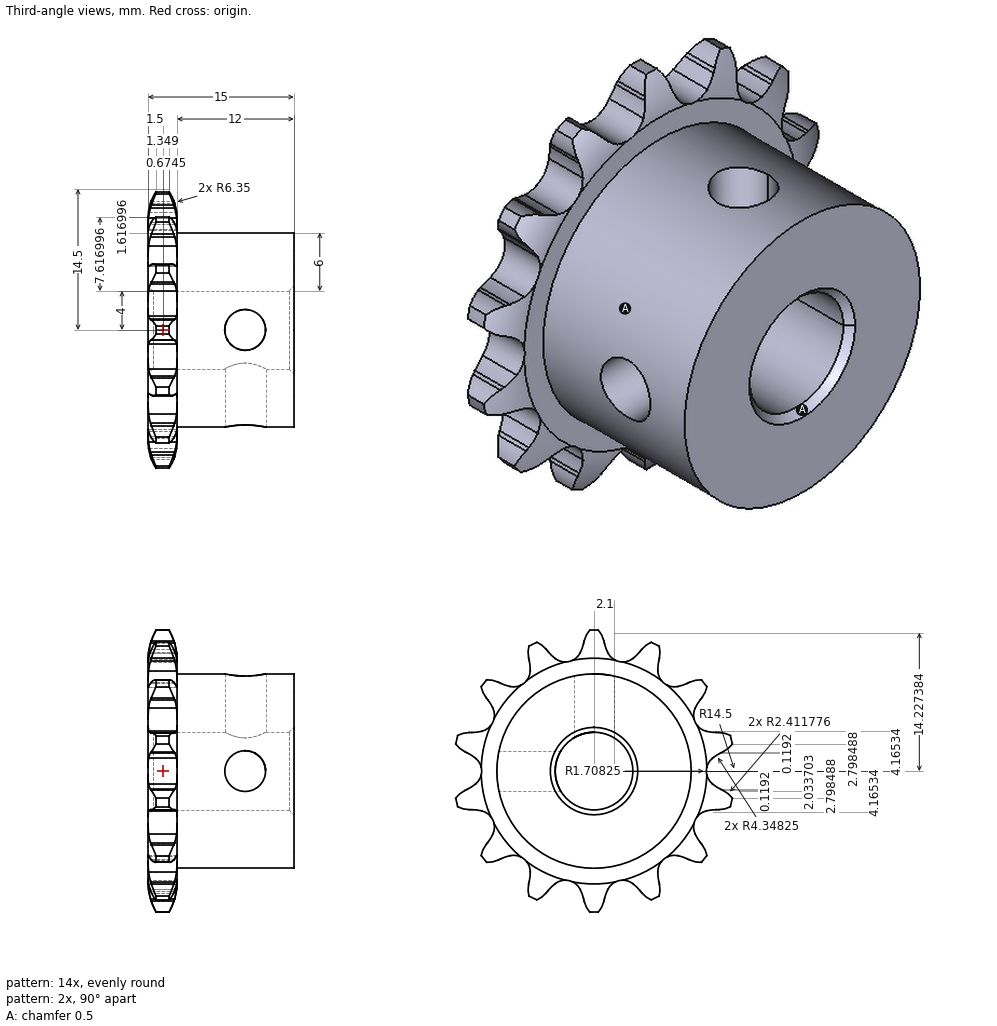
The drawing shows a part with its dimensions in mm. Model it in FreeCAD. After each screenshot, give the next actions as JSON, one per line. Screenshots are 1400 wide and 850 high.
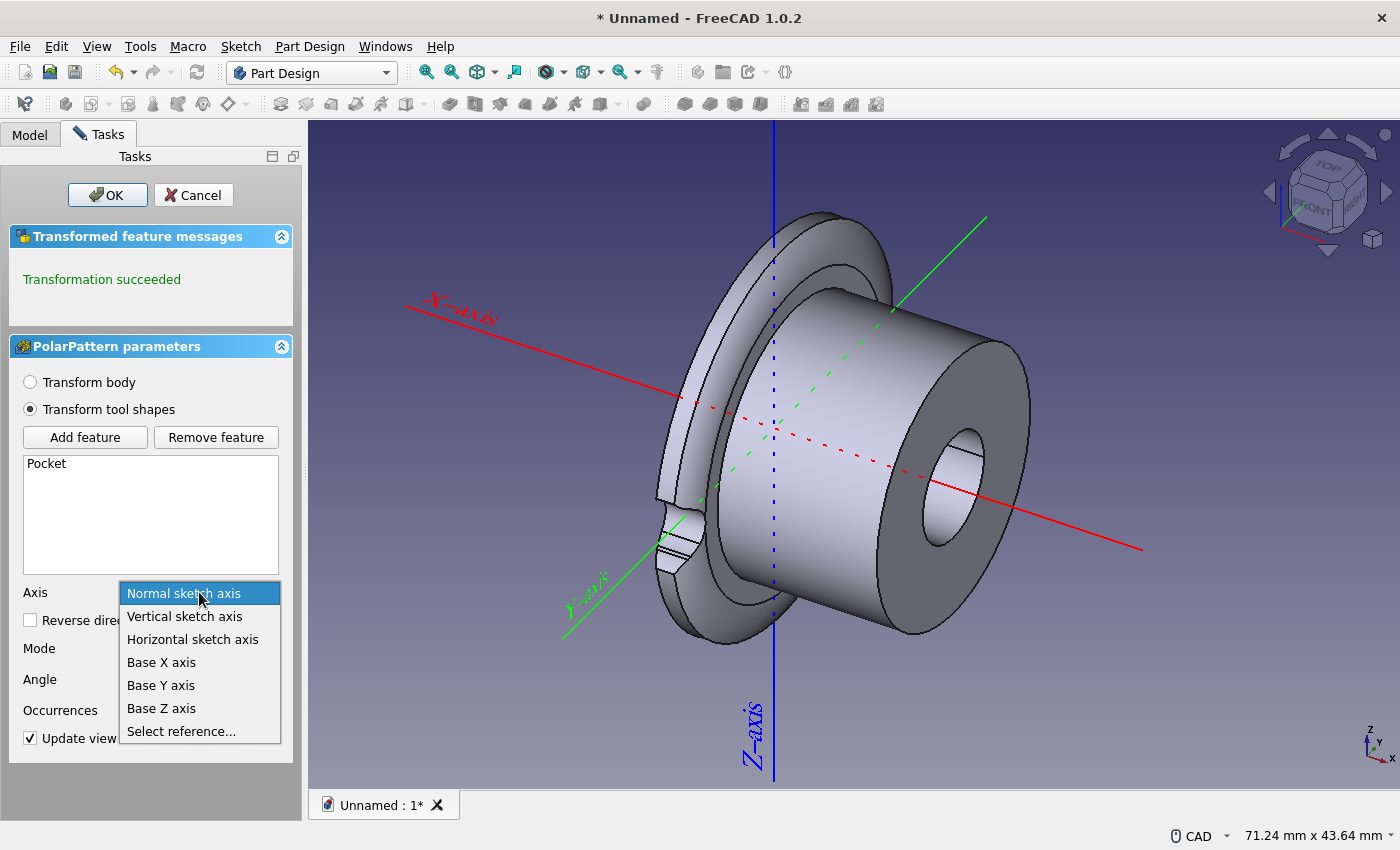
{"action": "left_click", "coordinate": [198, 662]}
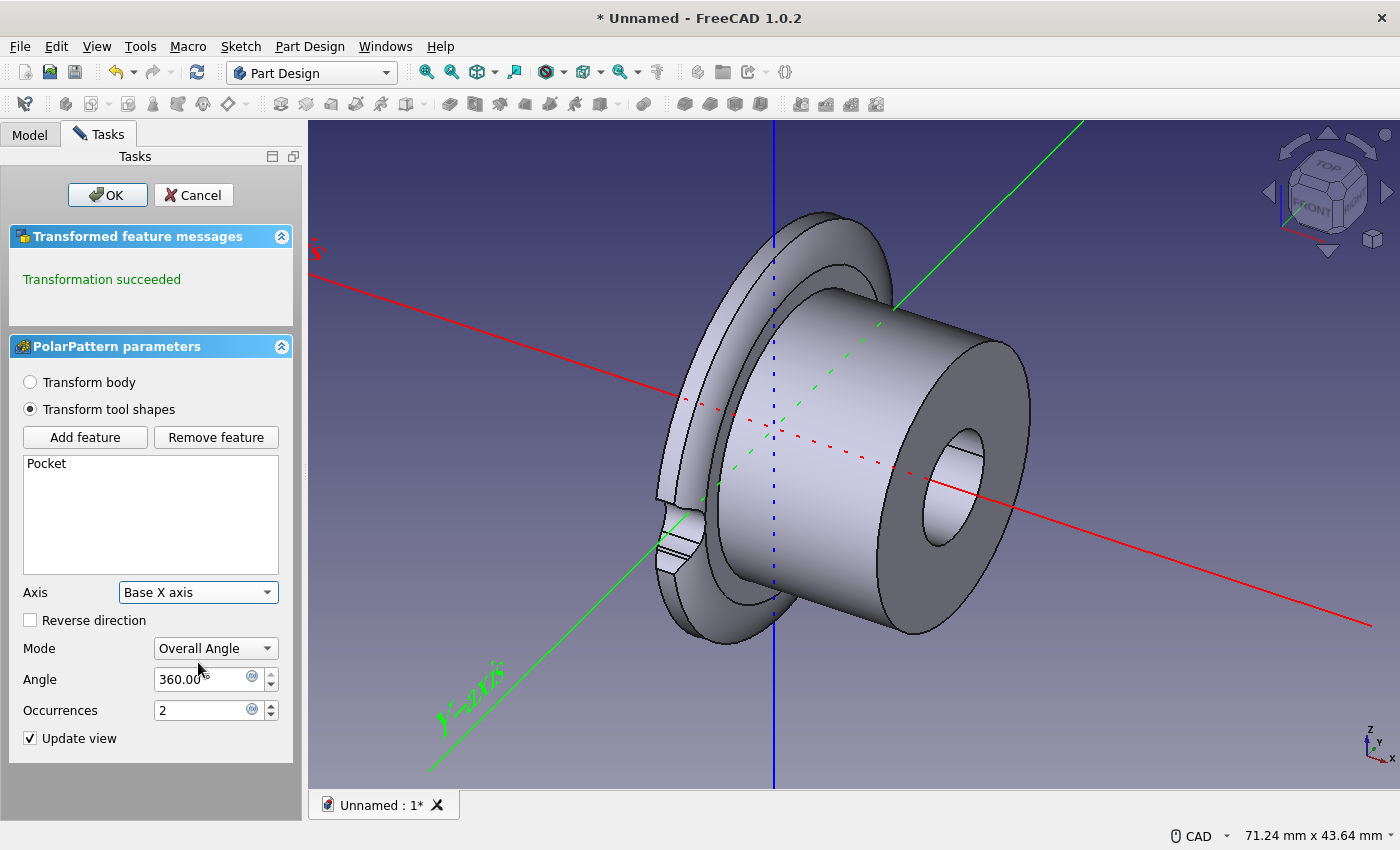
{"action": "triple_click", "coordinate": [210, 710]}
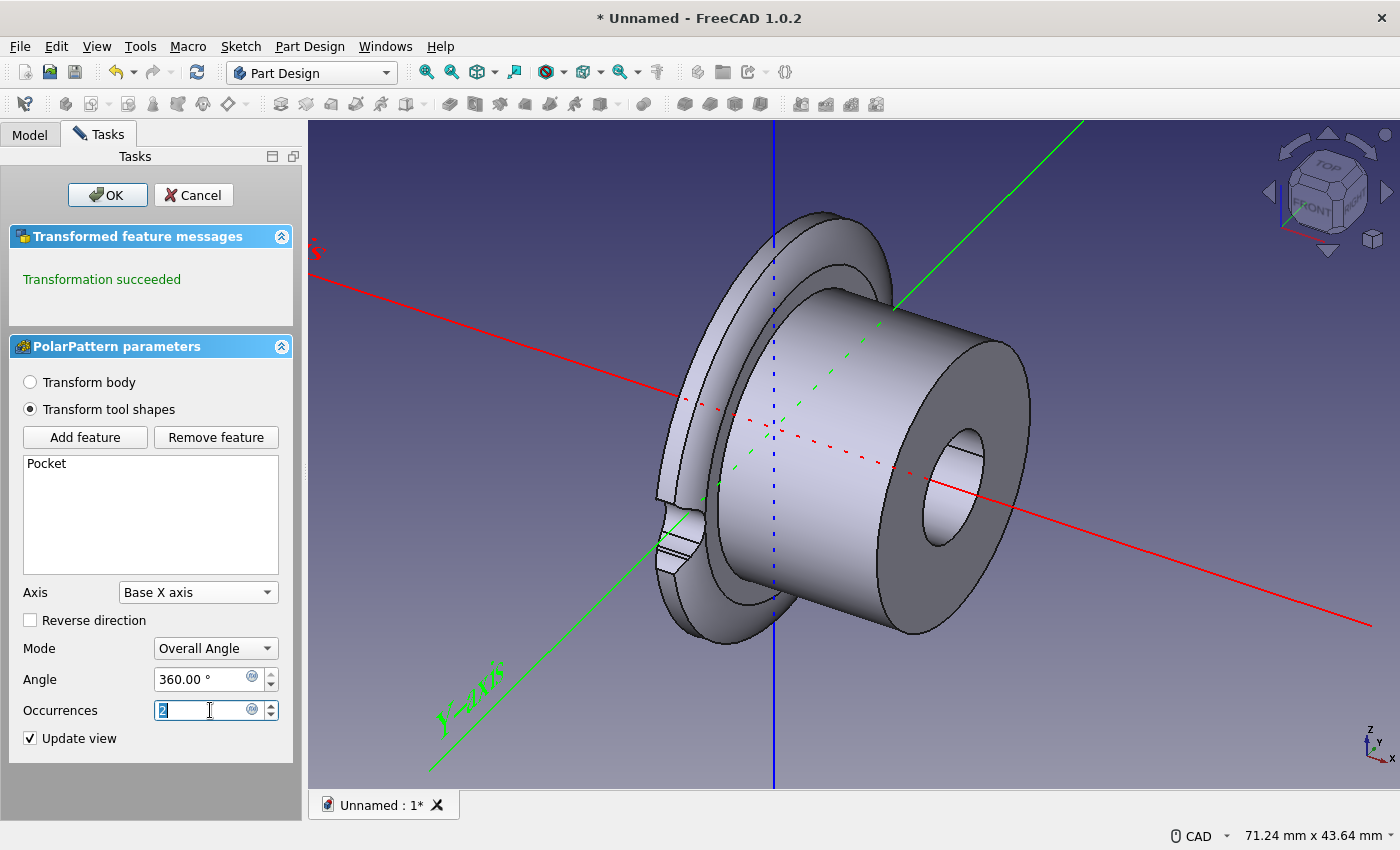
{"action": "type", "text": "14"}
{"action": "key", "text": "Tab"}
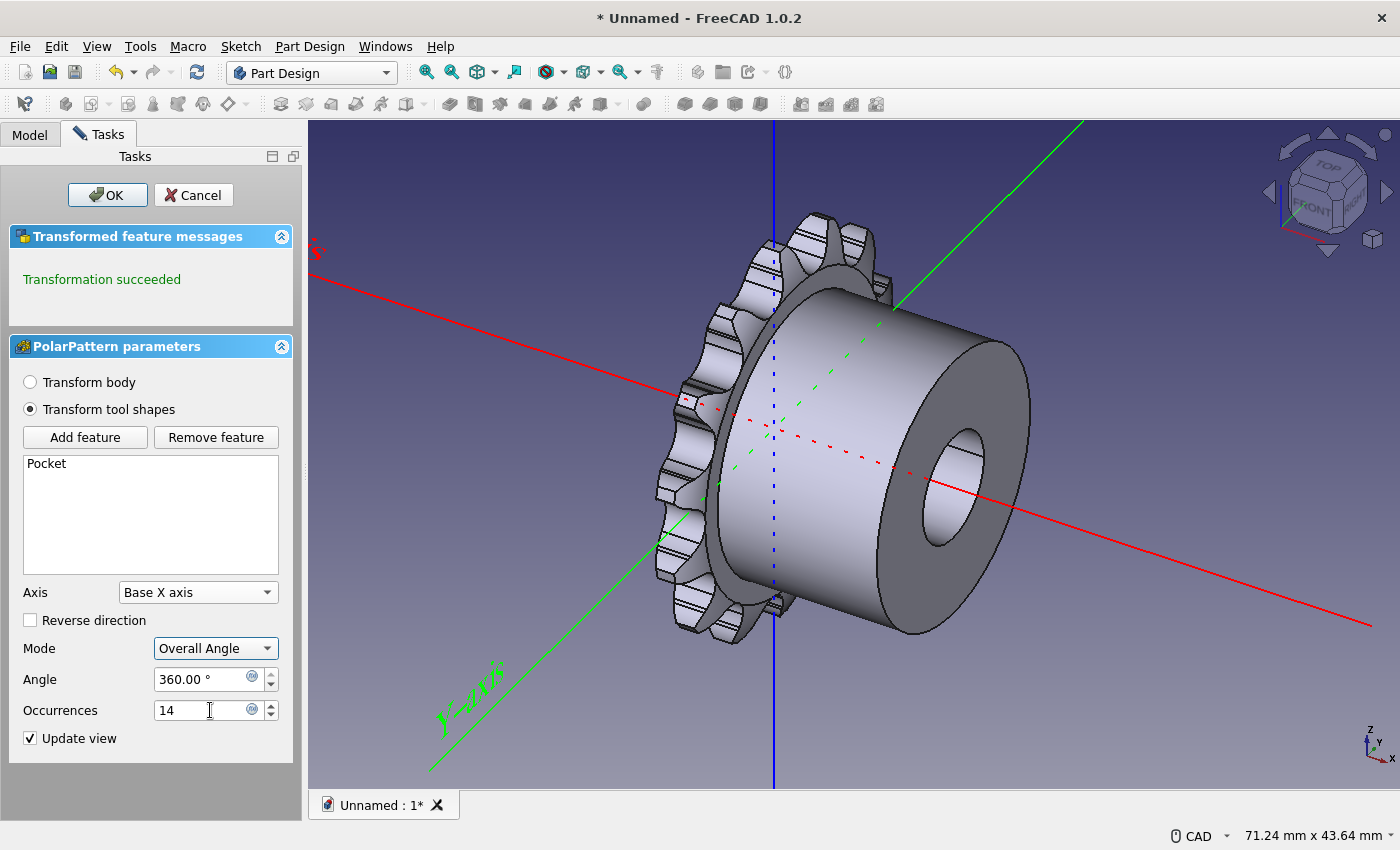
{"action": "left_click", "coordinate": [108, 195]}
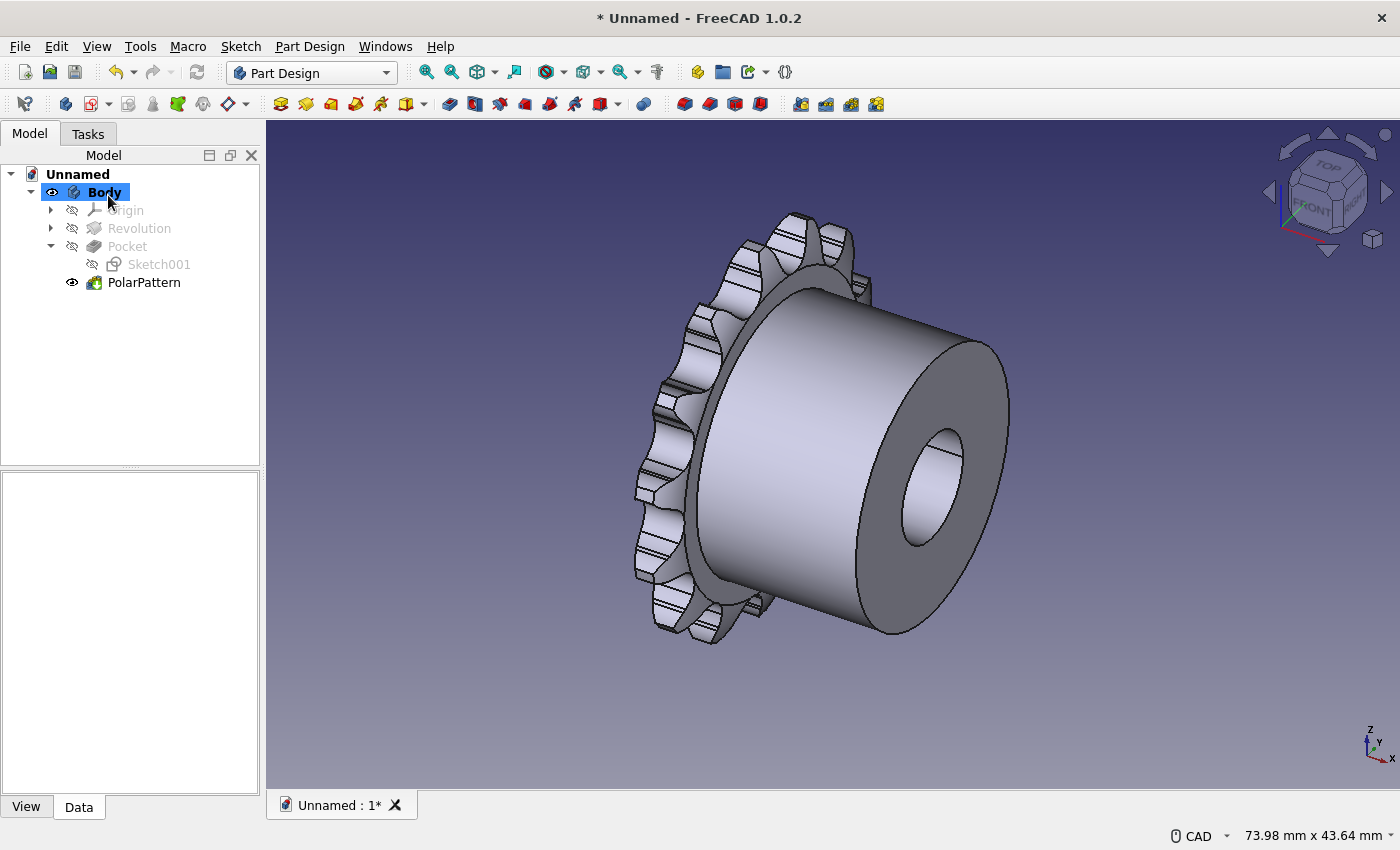
{"action": "left_click", "coordinate": [51, 210]}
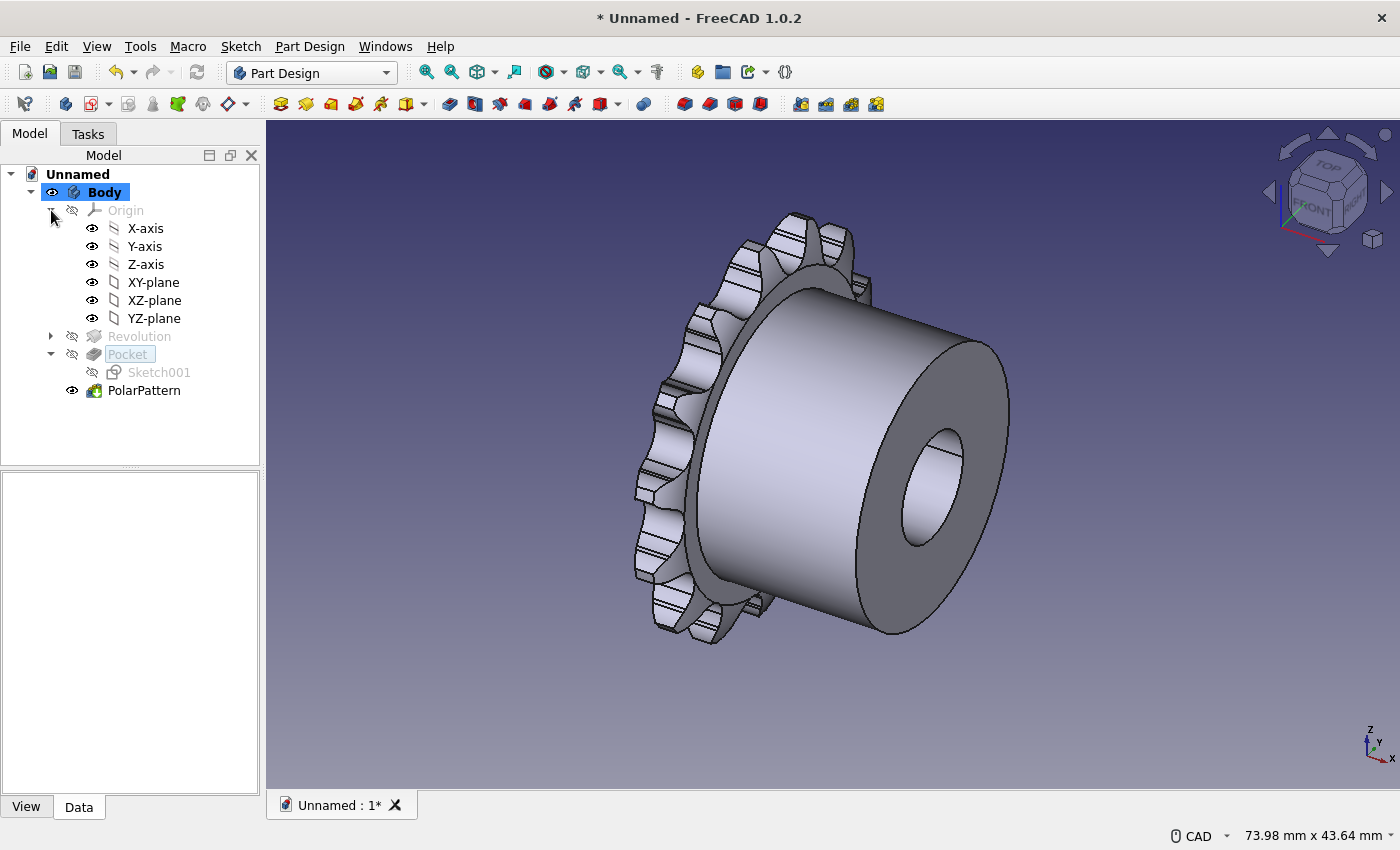
{"action": "left_click", "coordinate": [137, 318]}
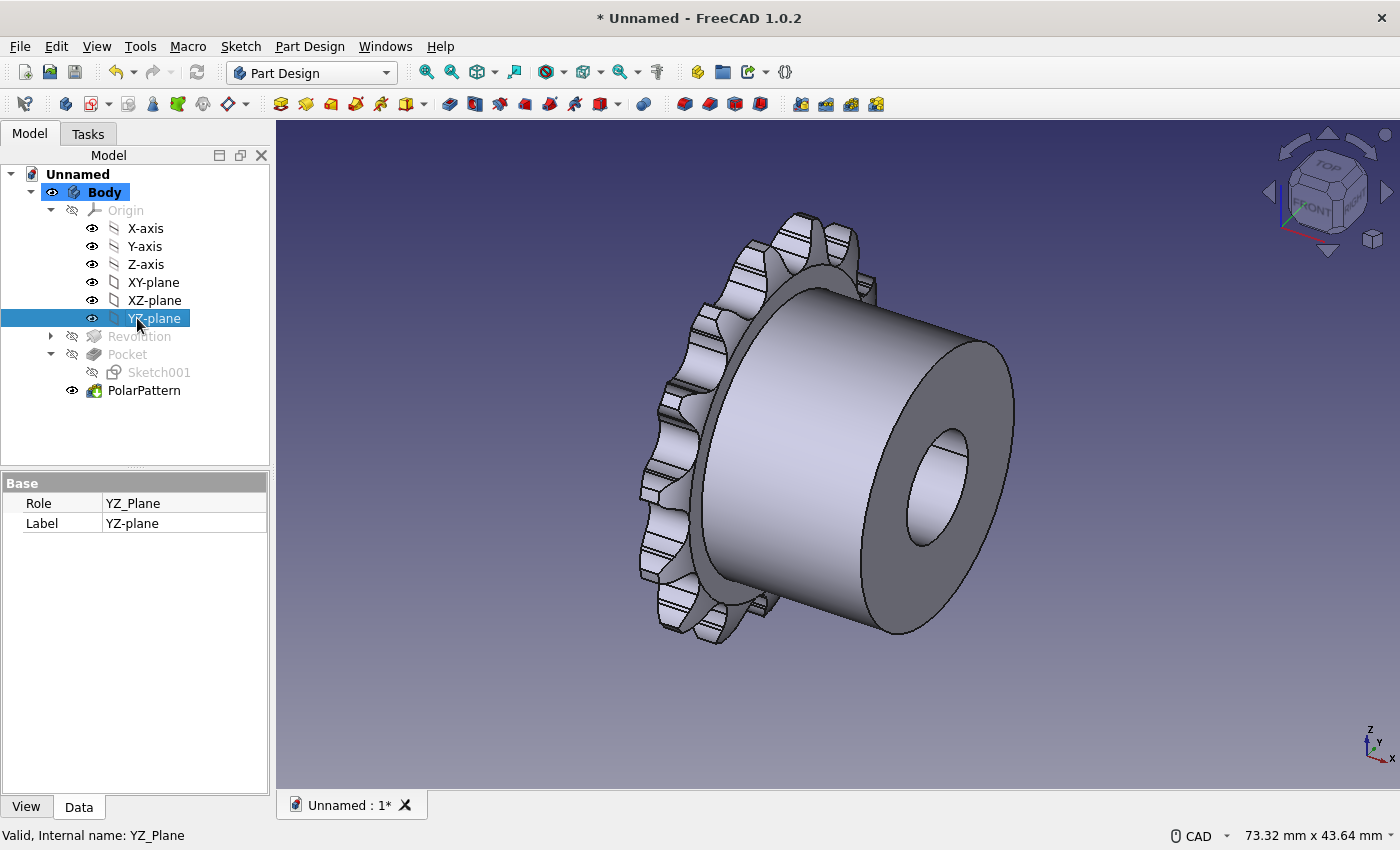
{"action": "left_click", "coordinate": [228, 104]}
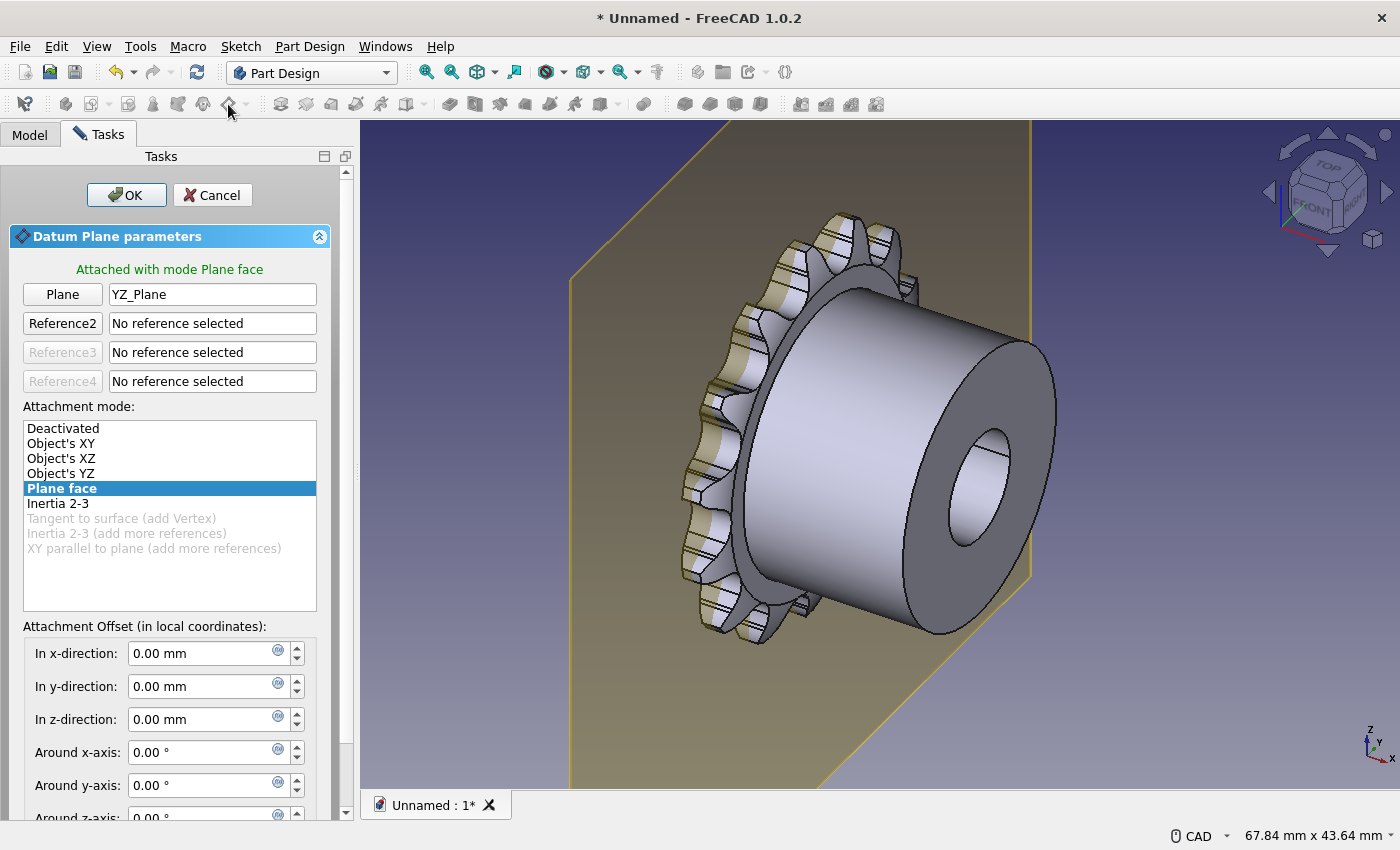
{"action": "triple_click", "coordinate": [210, 720]}